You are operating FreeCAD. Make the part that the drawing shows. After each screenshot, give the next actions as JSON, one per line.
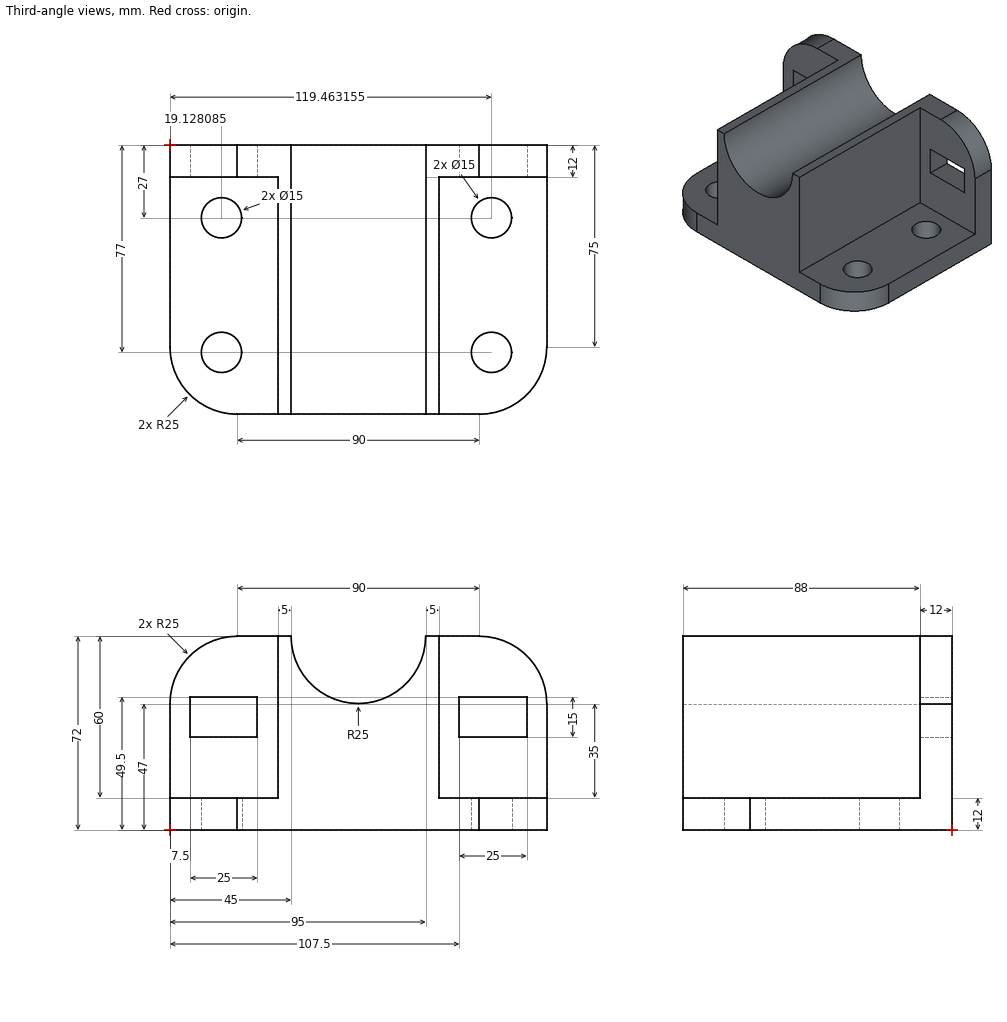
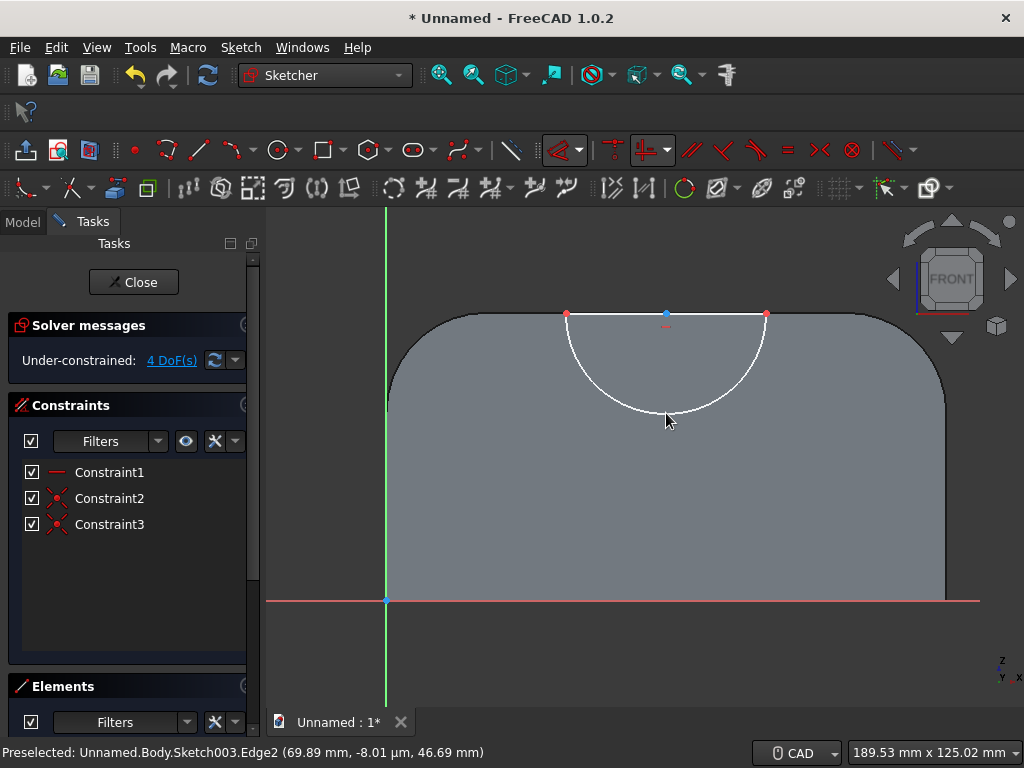
{"action": "left_click", "coordinate": [607, 395]}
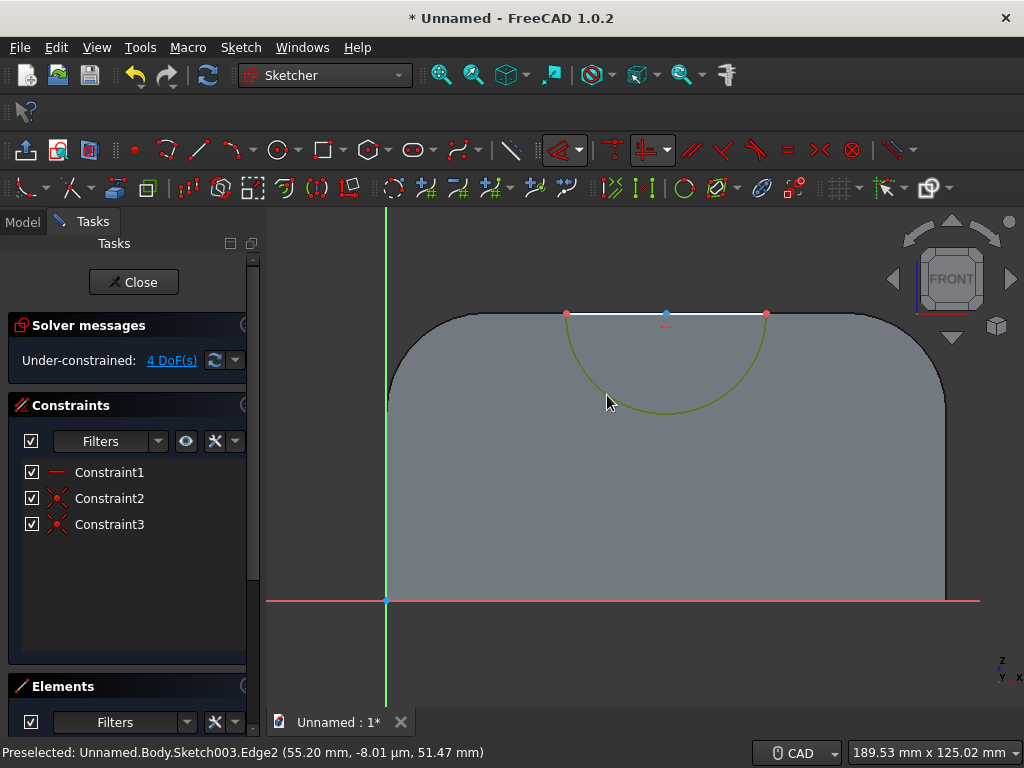
{"action": "key", "text": "k r"}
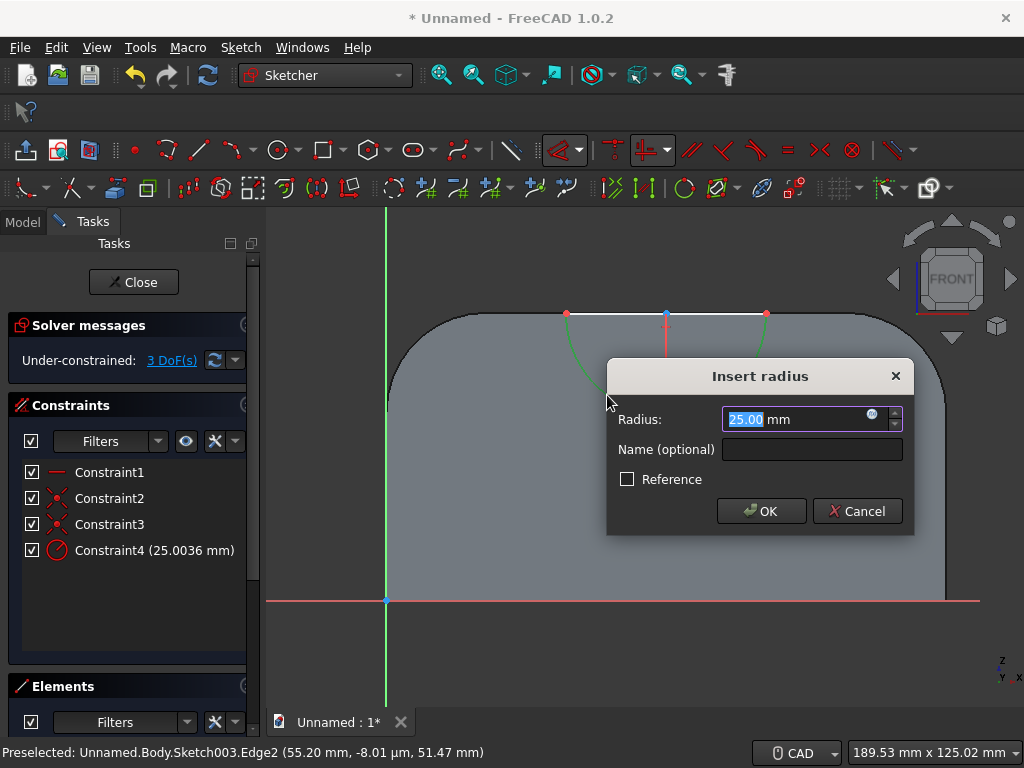
{"action": "type", "text": "25"}
{"action": "key", "text": "Return"}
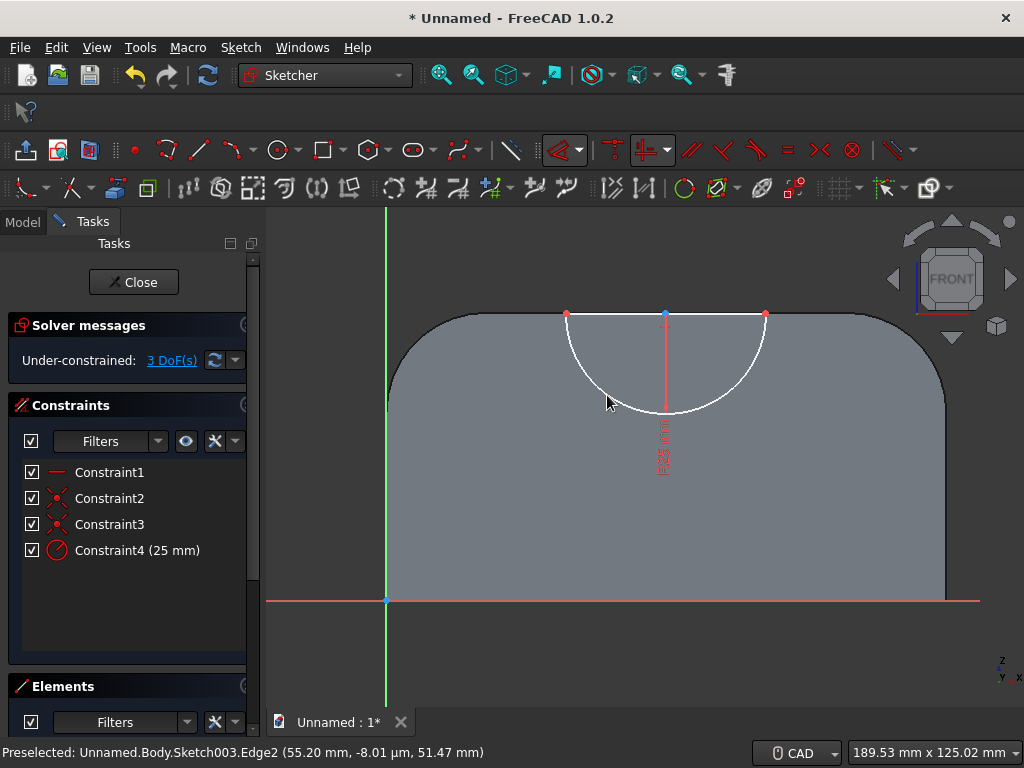
{"action": "left_click", "coordinate": [766, 314]}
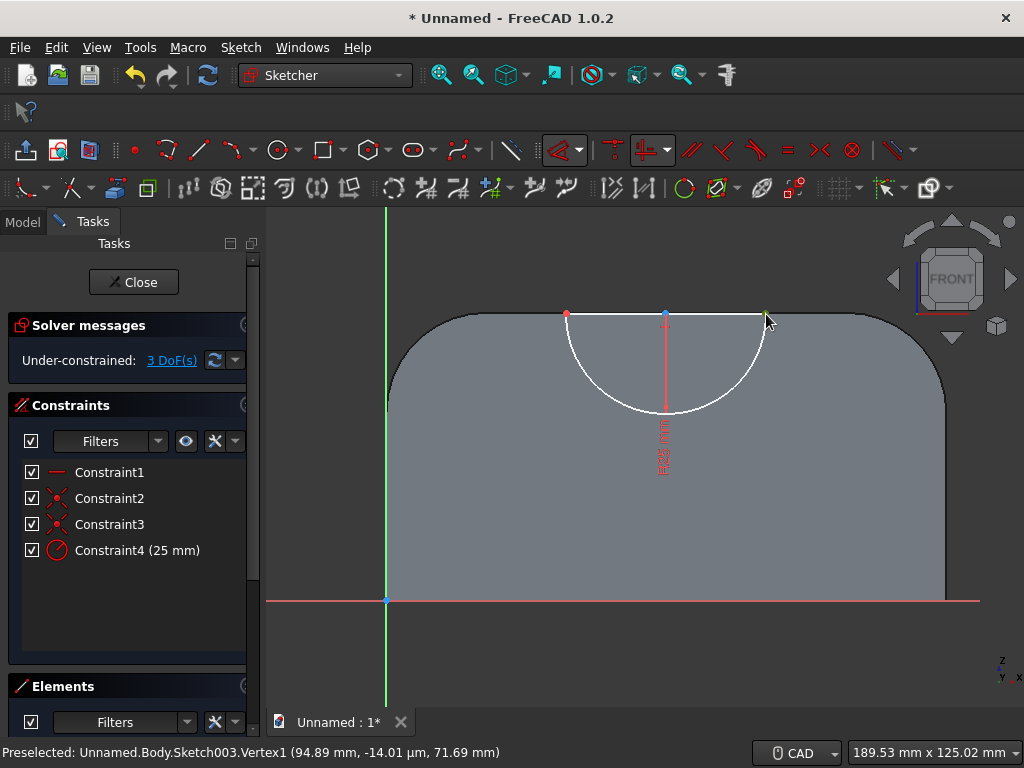
{"action": "key", "text": "l"}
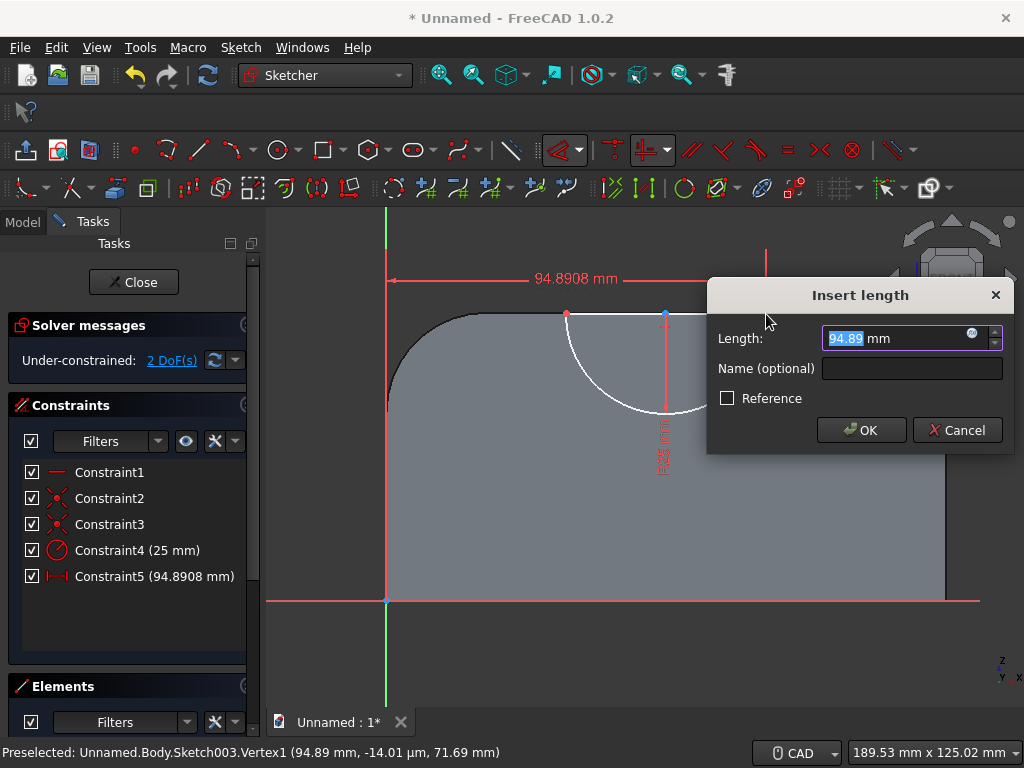
{"action": "type", "text": "95"}
{"action": "key", "text": "Return"}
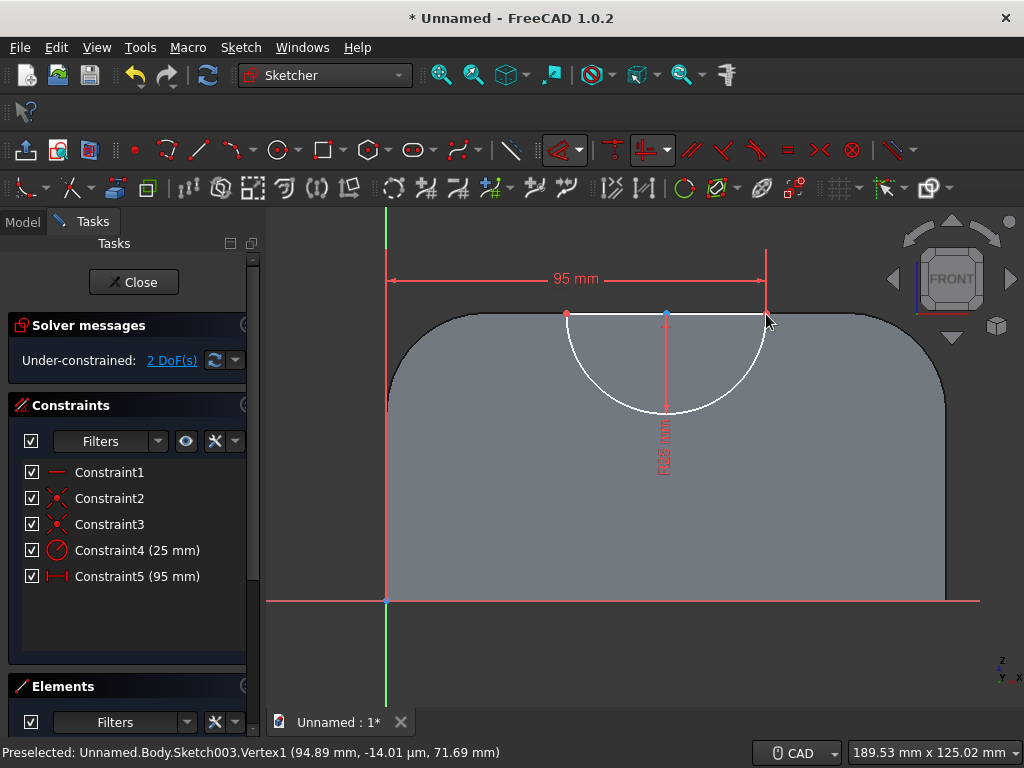
{"action": "left_click", "coordinate": [766, 314]}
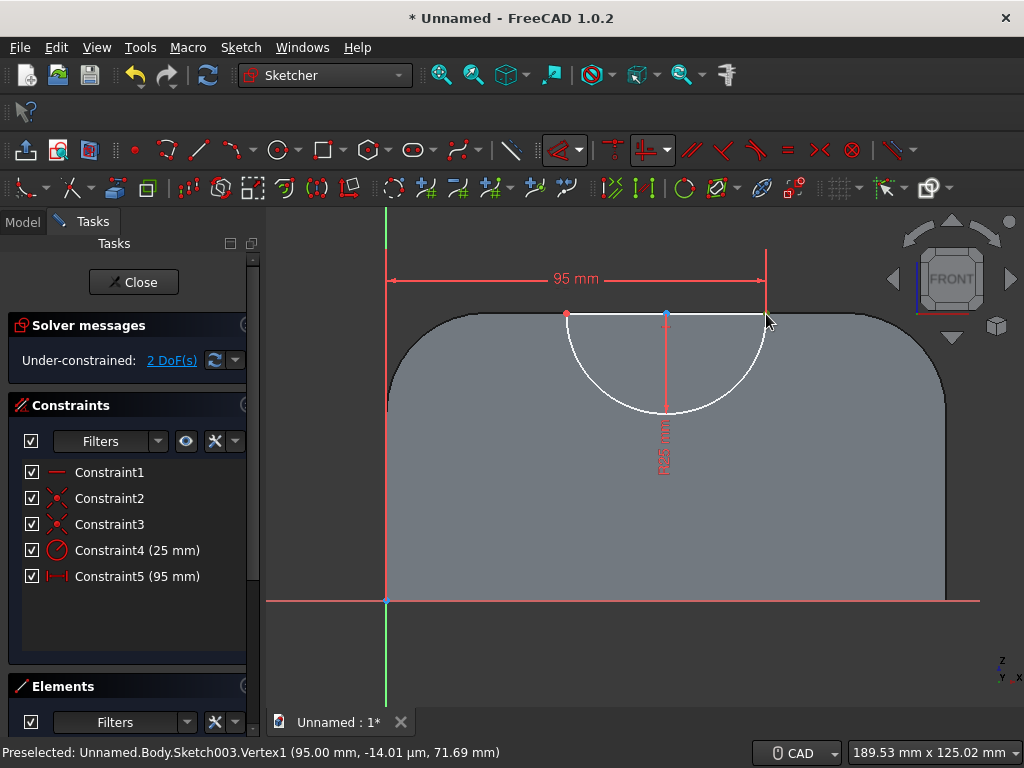
{"action": "key", "text": "i"}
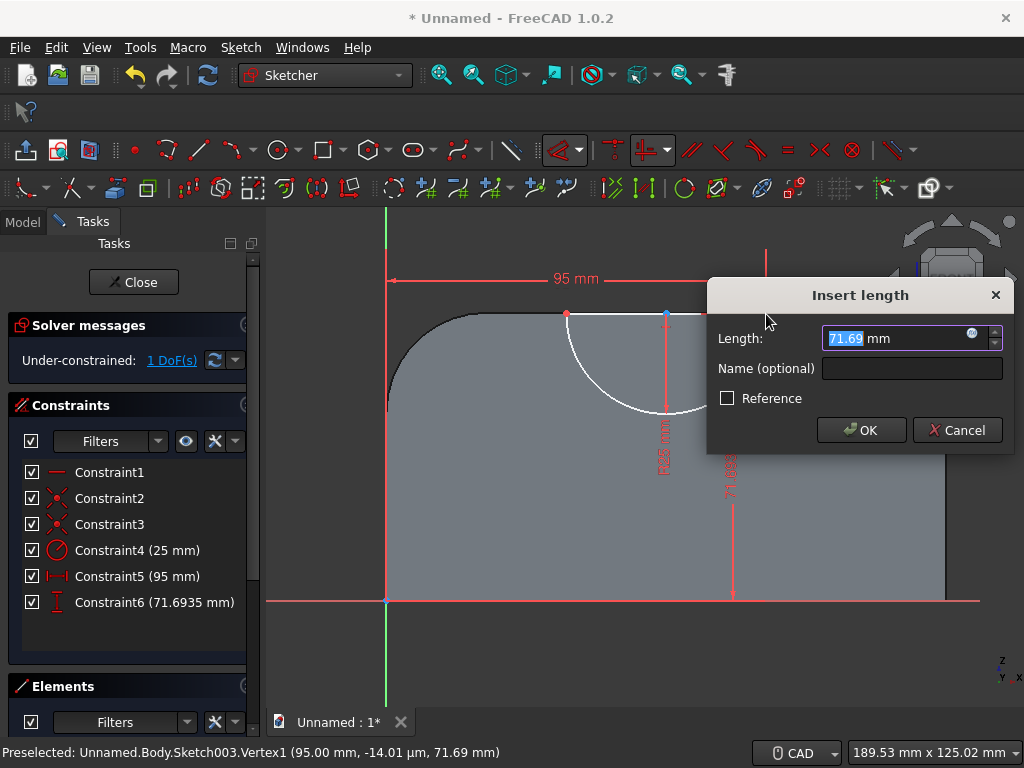
{"action": "type", "text": "72"}
{"action": "key", "text": "Return"}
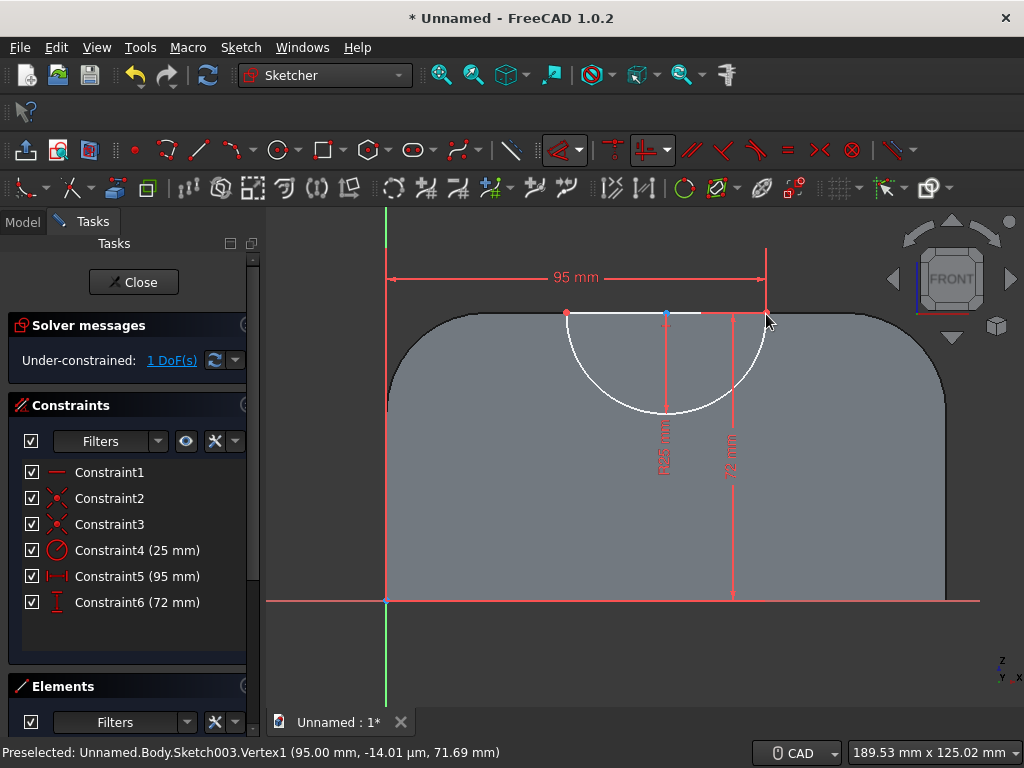
{"action": "left_click", "coordinate": [666, 314]}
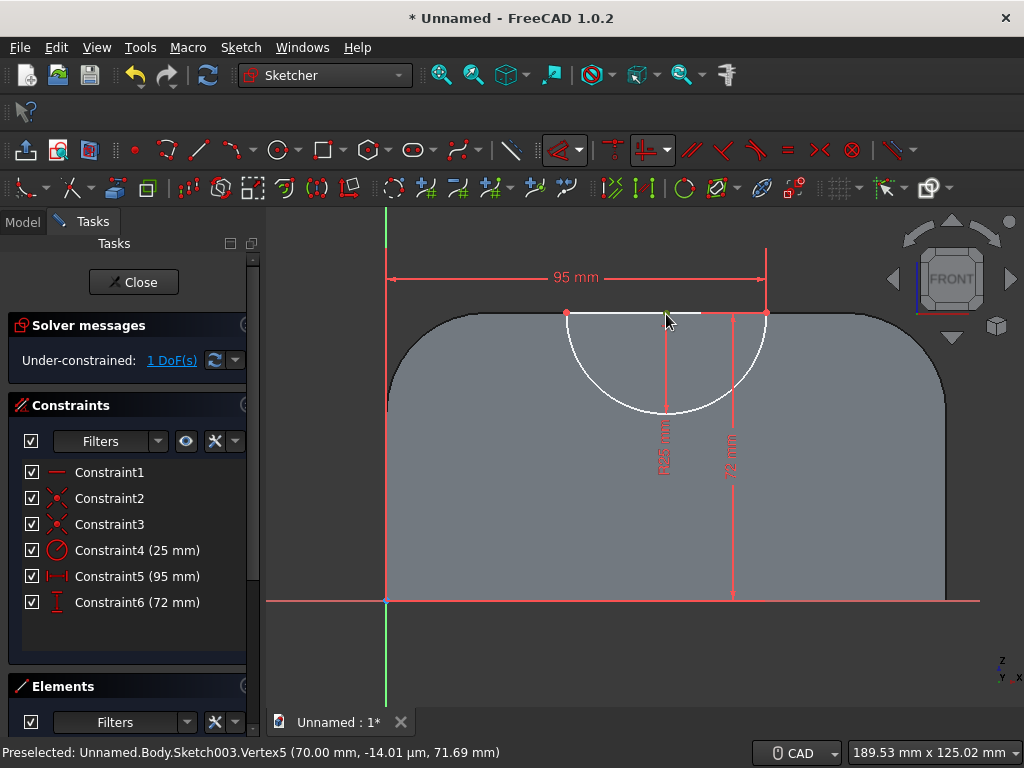
{"action": "key", "text": "i"}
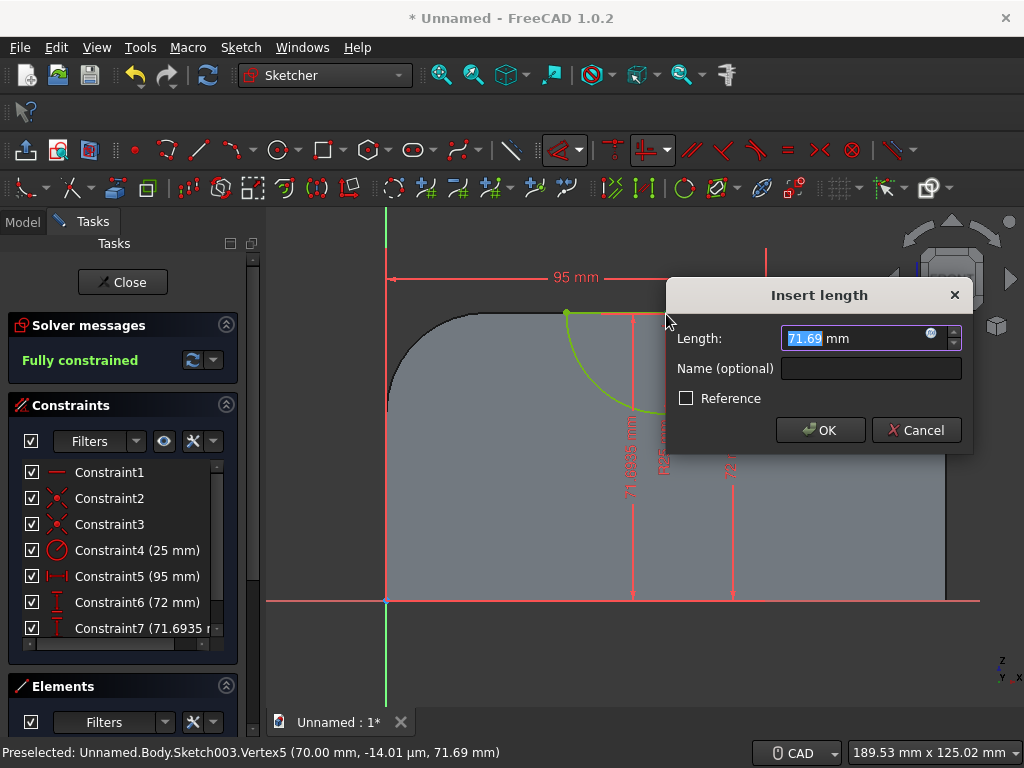
{"action": "type", "text": "72"}
{"action": "key", "text": "Return"}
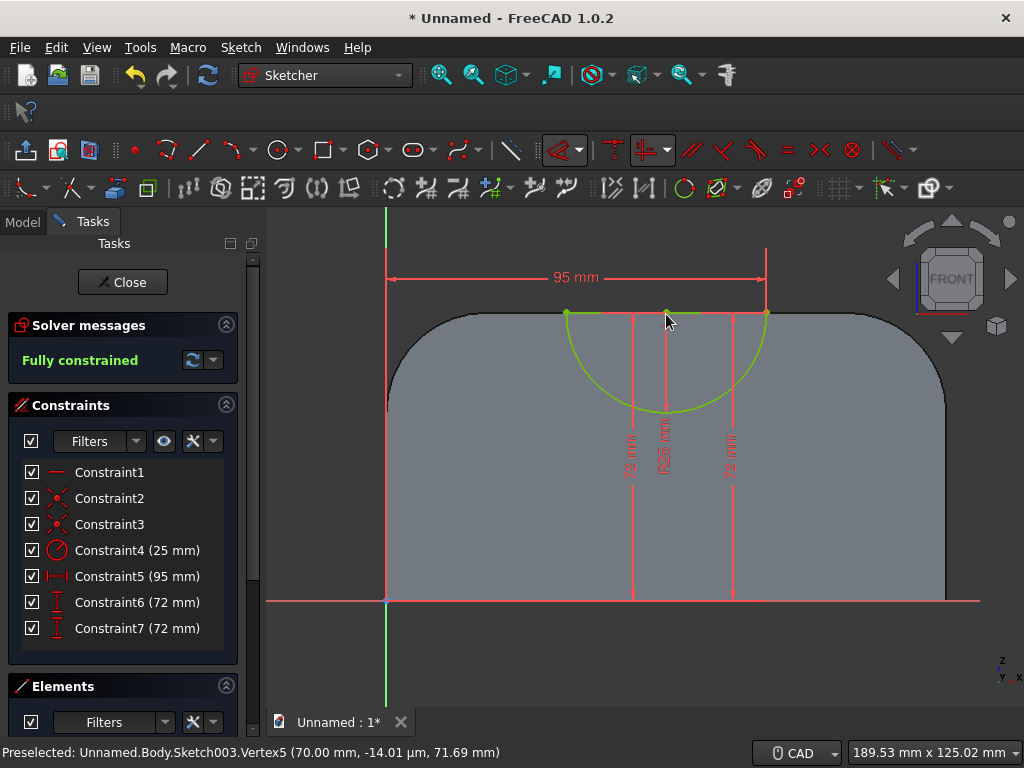
{"action": "left_click", "coordinate": [123, 282]}